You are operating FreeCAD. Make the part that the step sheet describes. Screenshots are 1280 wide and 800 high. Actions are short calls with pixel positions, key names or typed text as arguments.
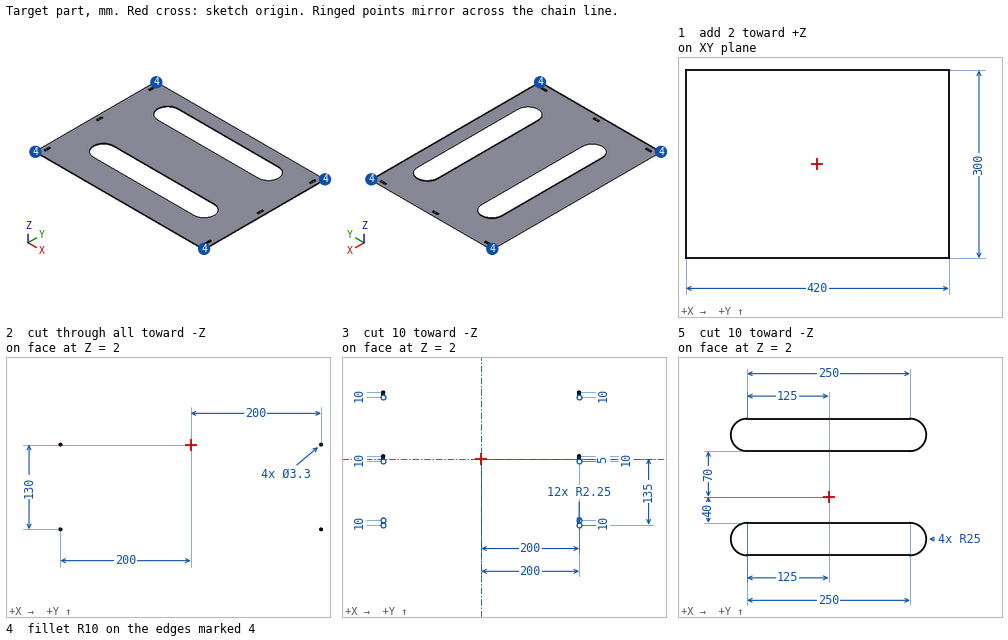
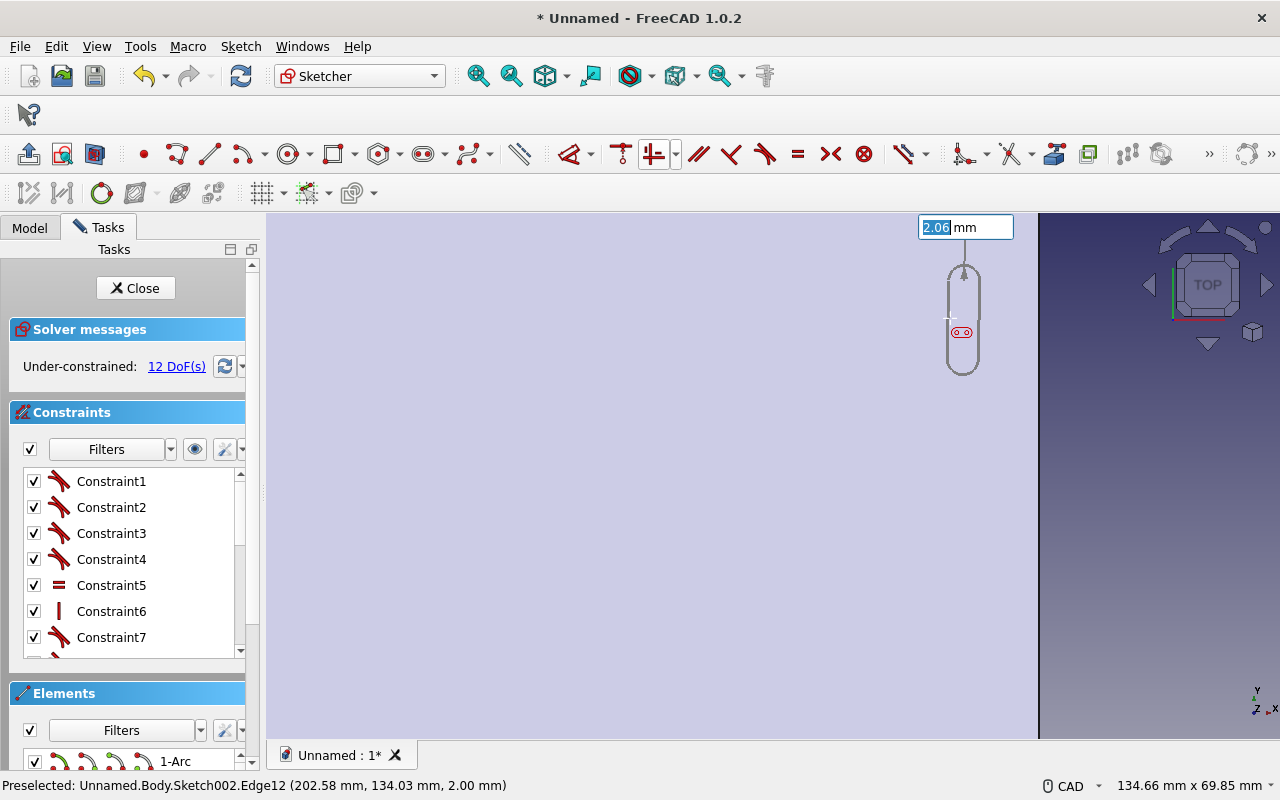
click(947, 315)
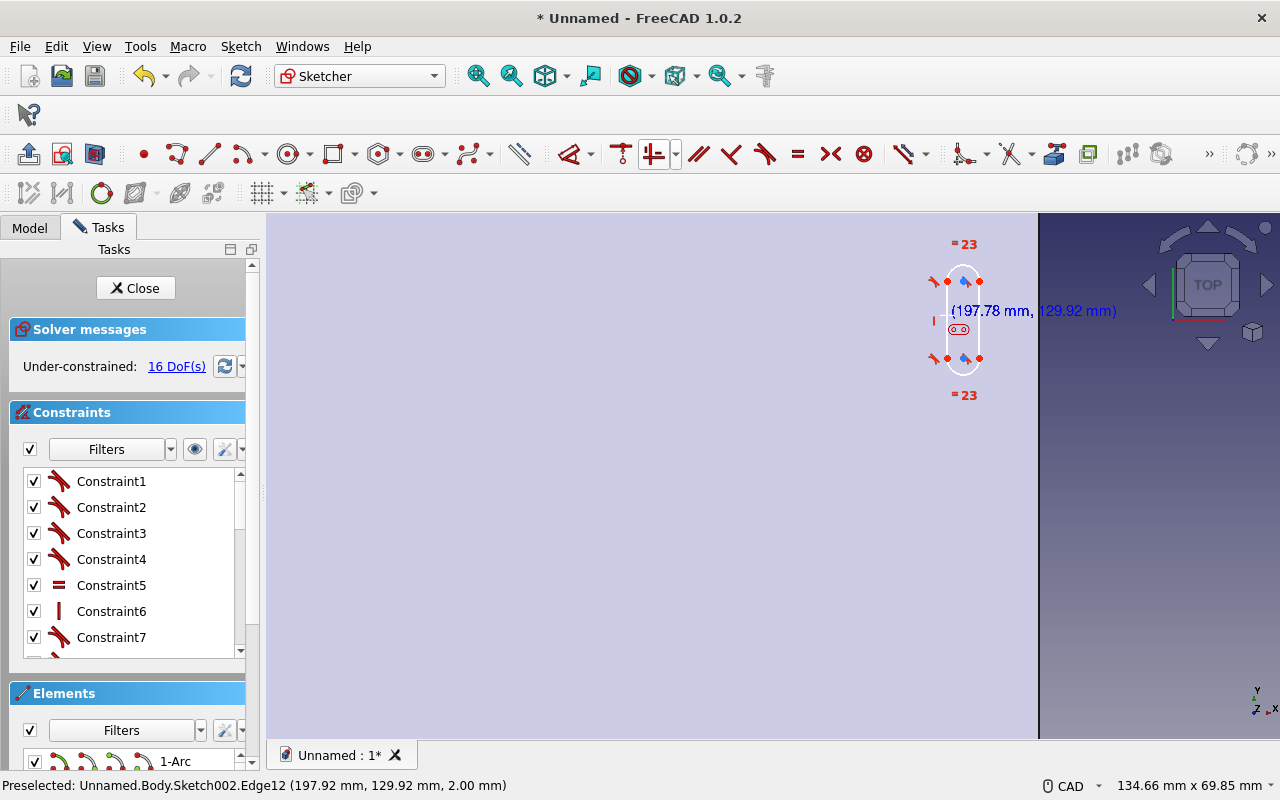
scroll(951, 314, down, 9)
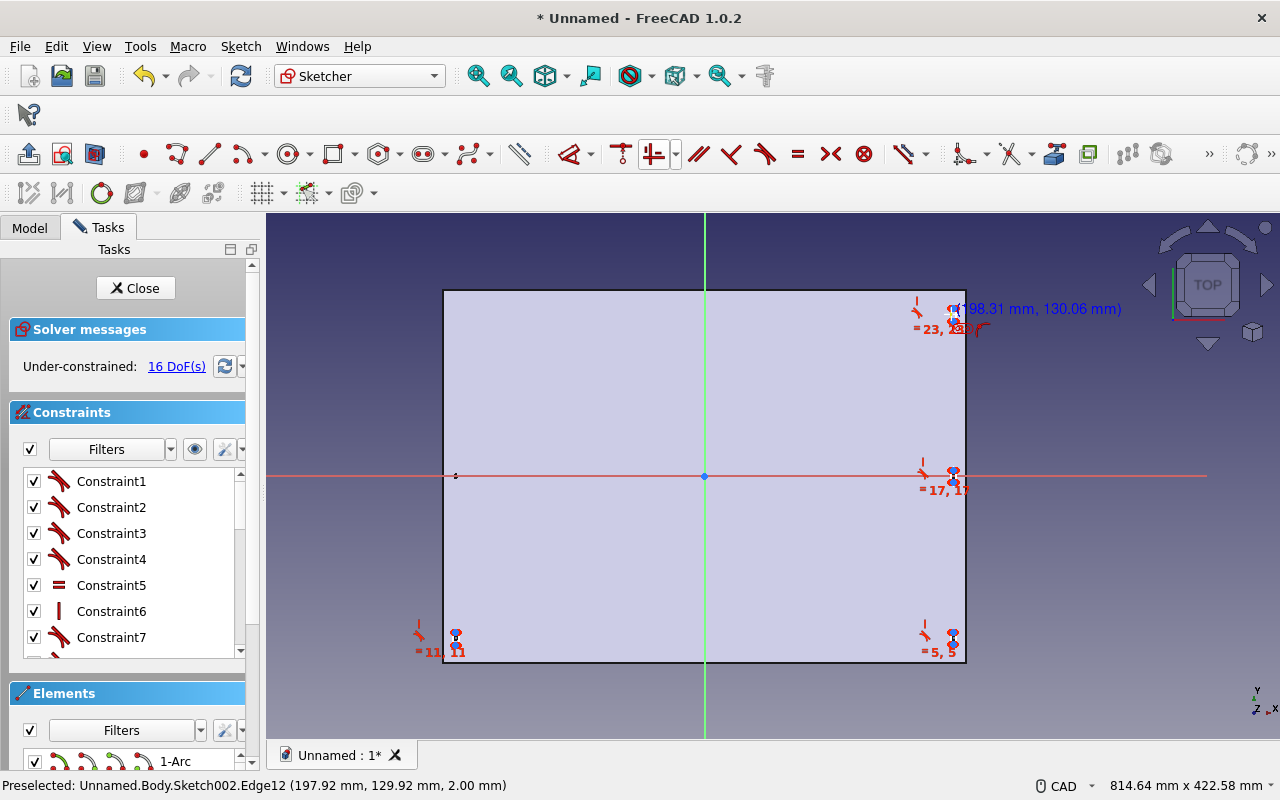
scroll(456, 321, up, 11)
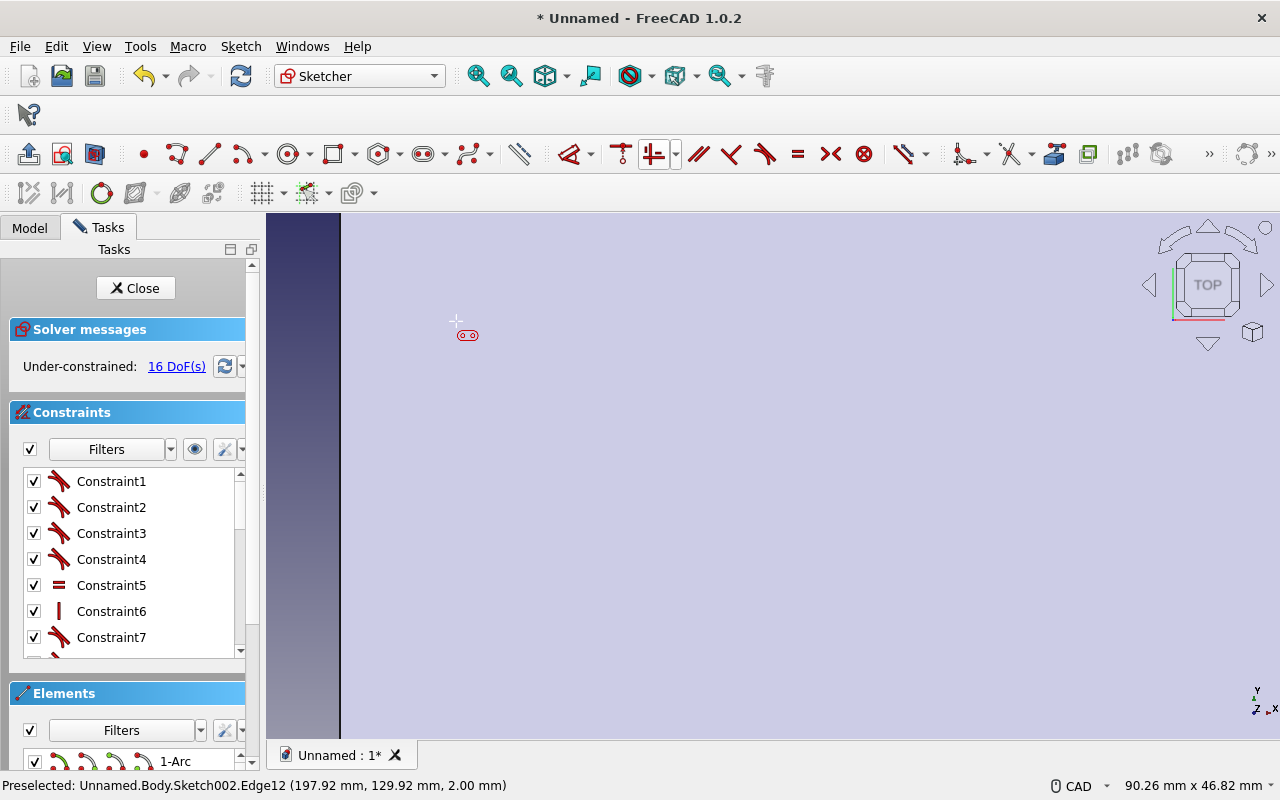
scroll(456, 321, down, 11)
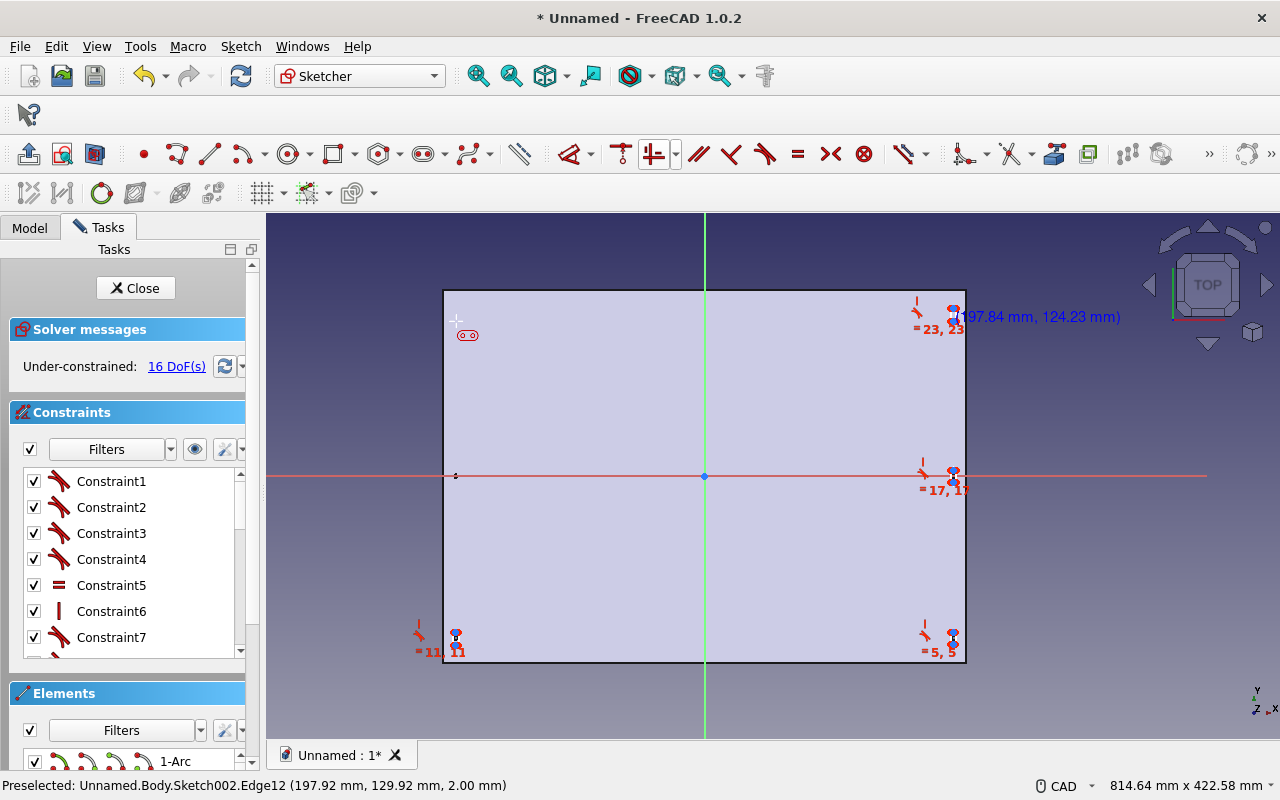
click(456, 321)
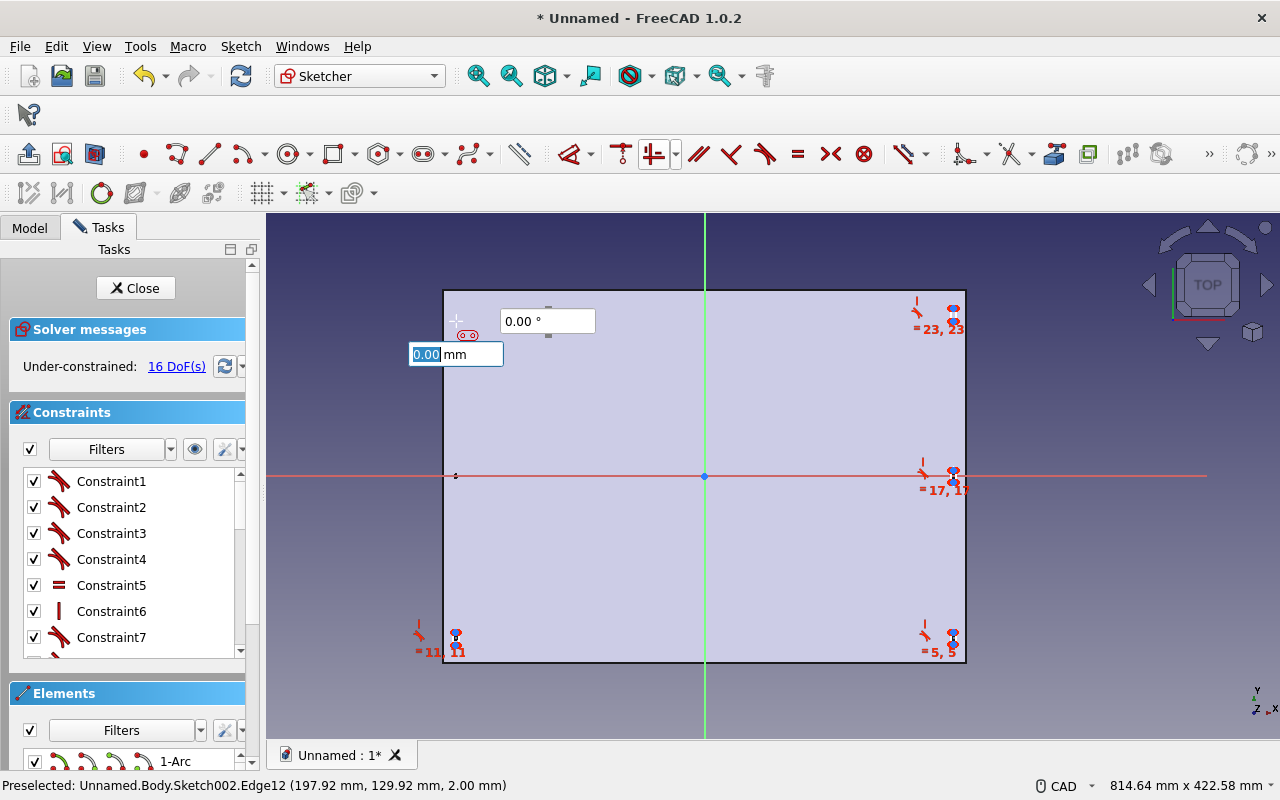
scroll(456, 308, up, 2)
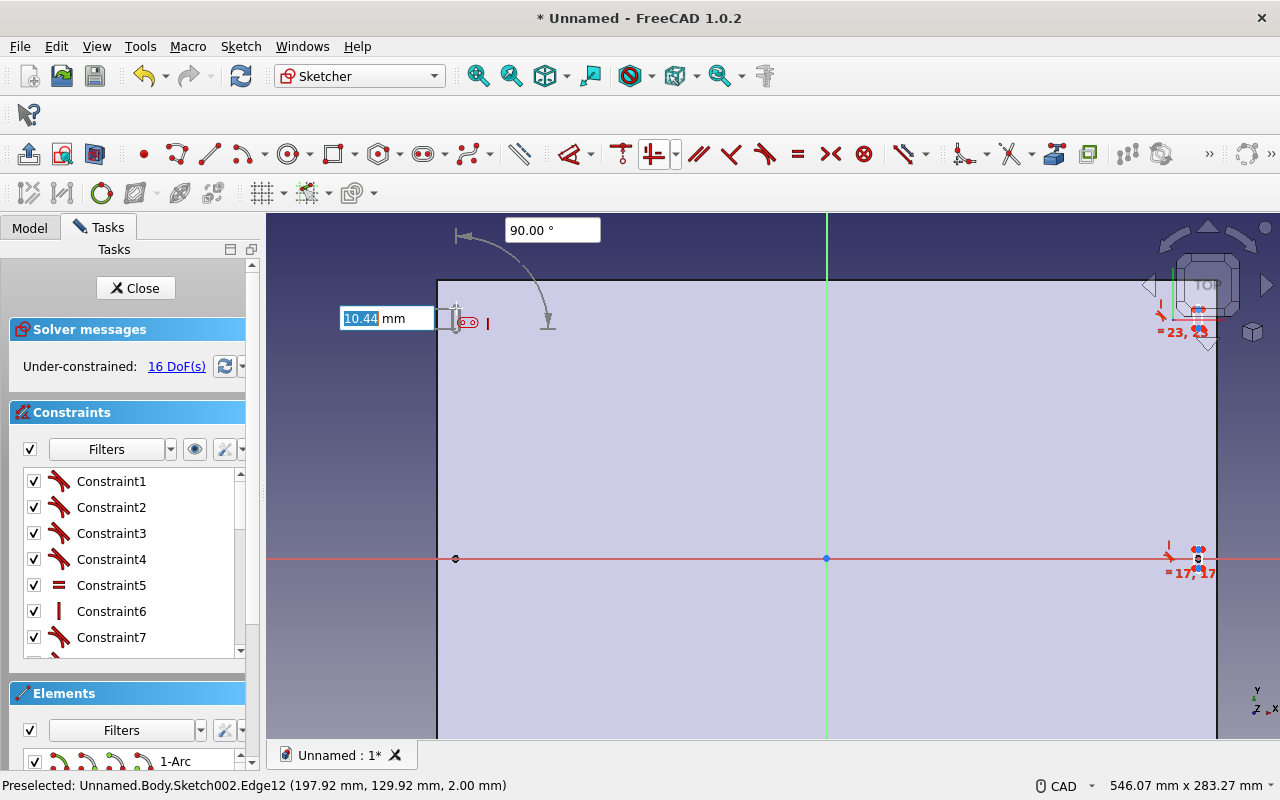
click(456, 308)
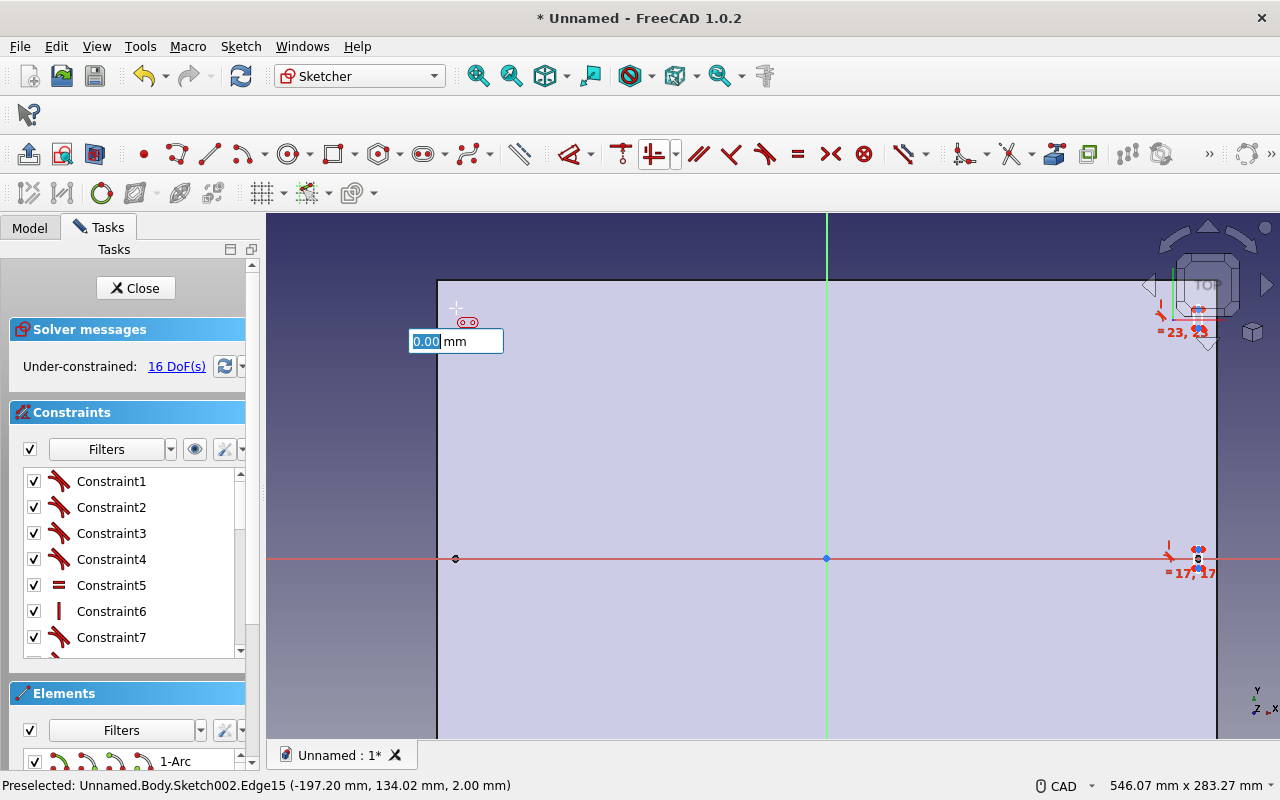
scroll(460, 317, up, 7)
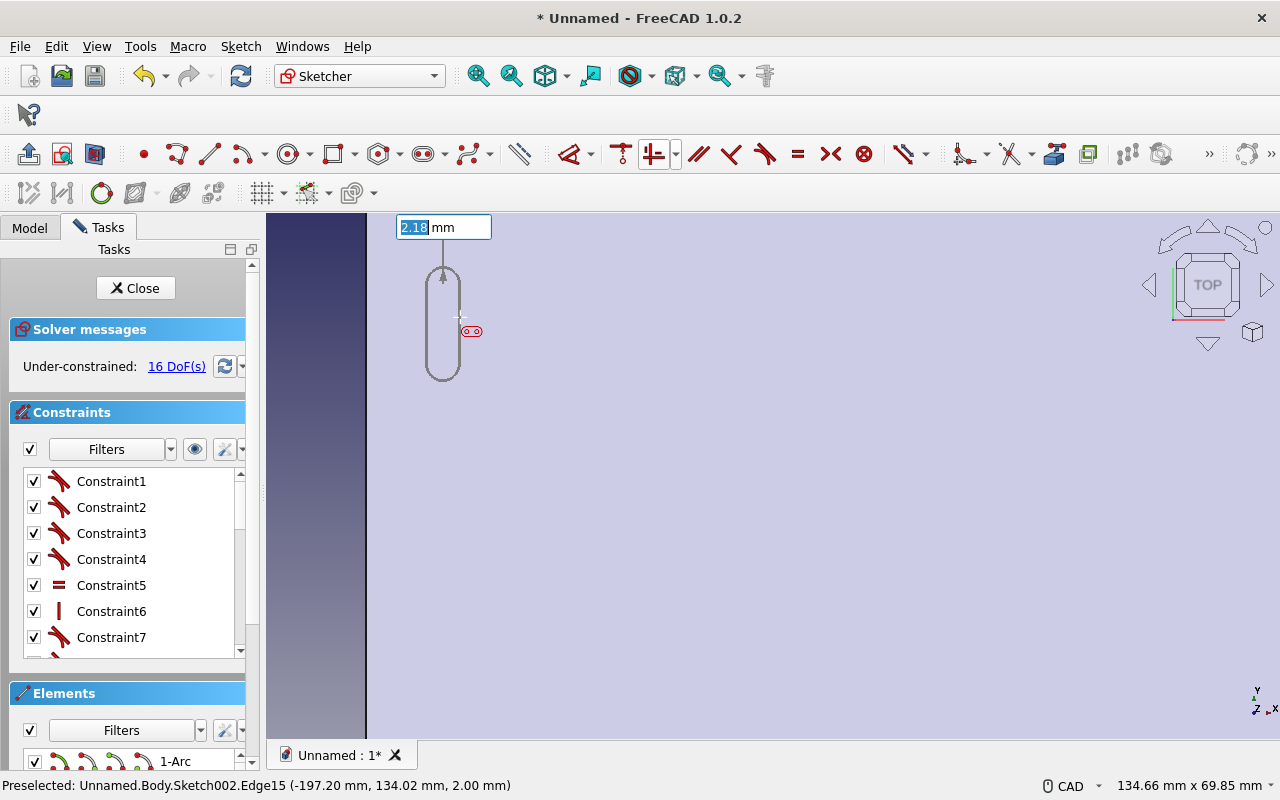
click(458, 318)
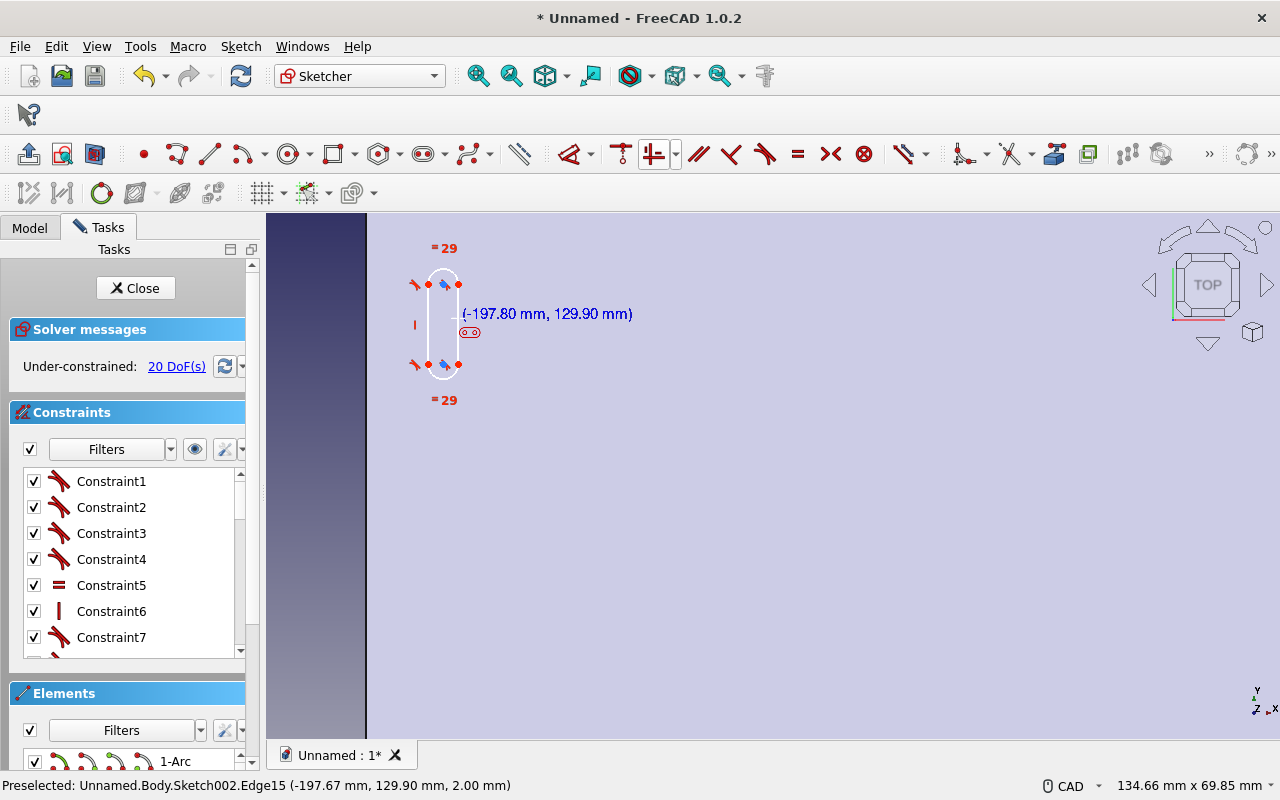
scroll(458, 313, down, 9)